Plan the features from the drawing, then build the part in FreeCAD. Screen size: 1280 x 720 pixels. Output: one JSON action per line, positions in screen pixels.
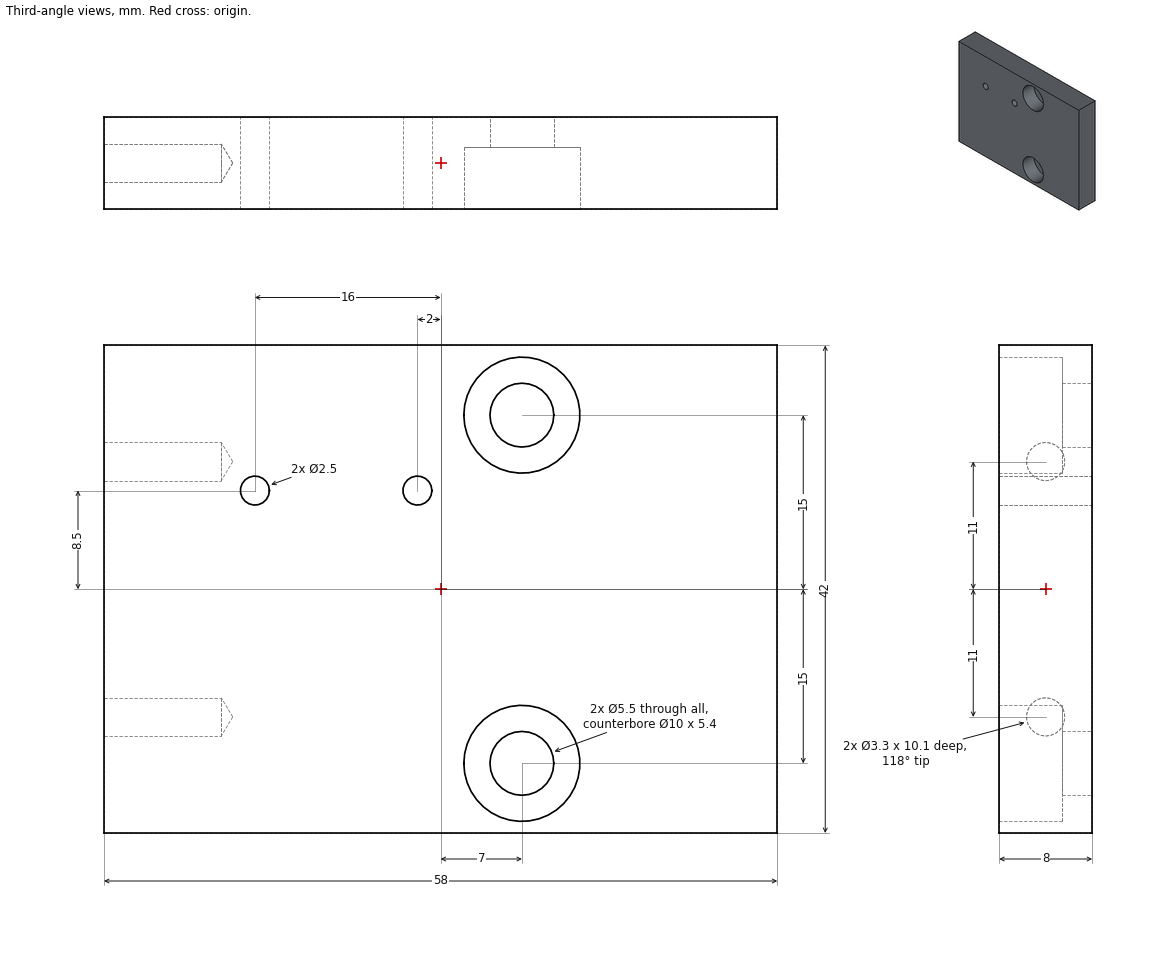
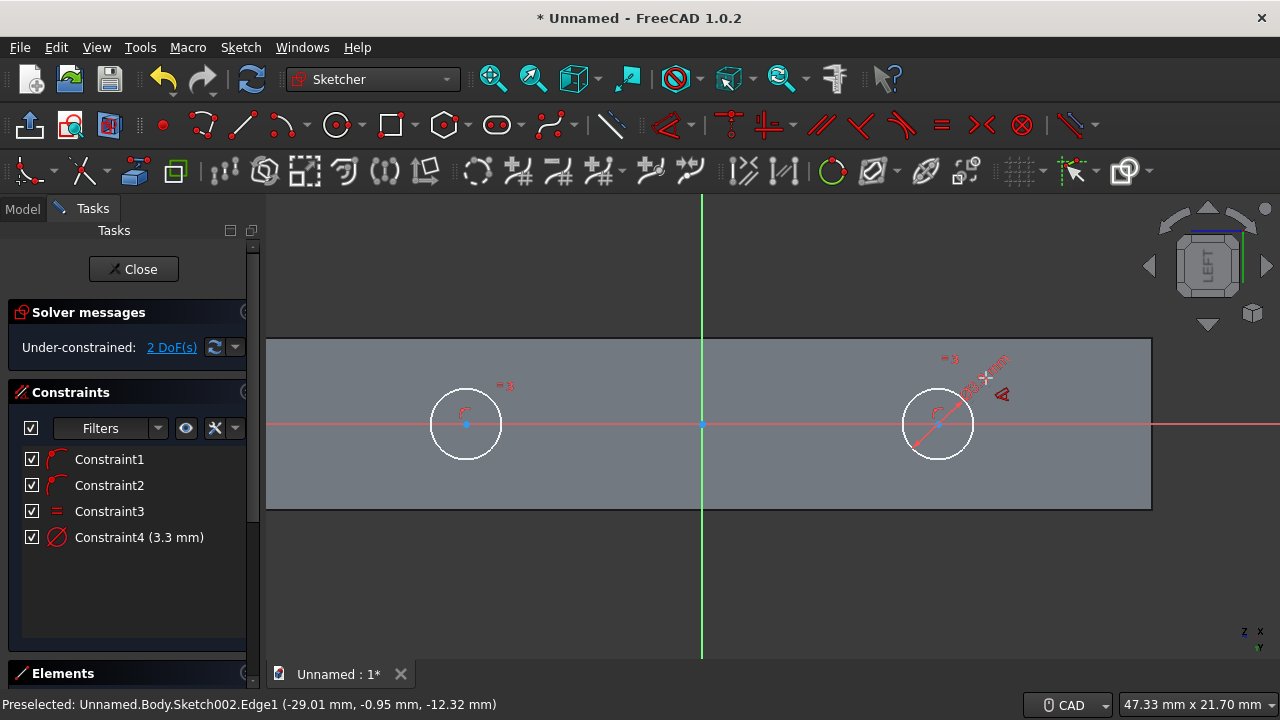
{"action": "left_click", "coordinate": [938, 424]}
{"action": "left_click", "coordinate": [820, 458]}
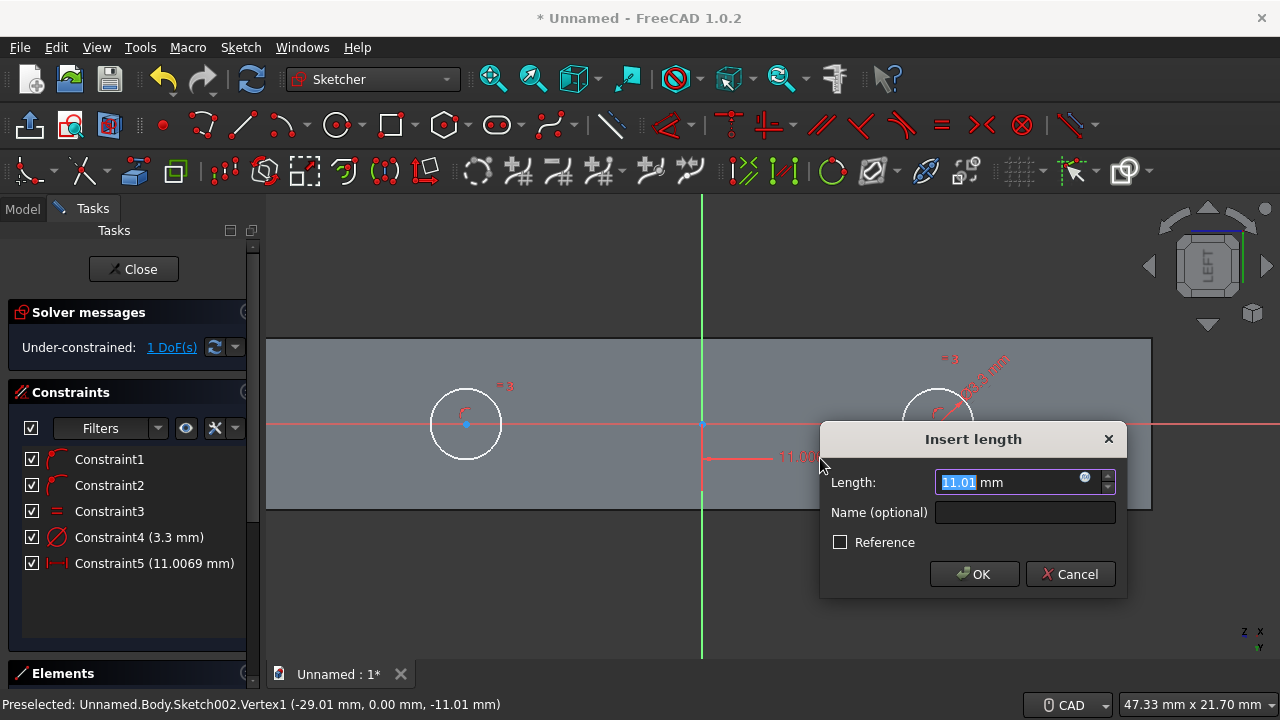
{"action": "type", "text": "11"}
{"action": "key", "text": "Return"}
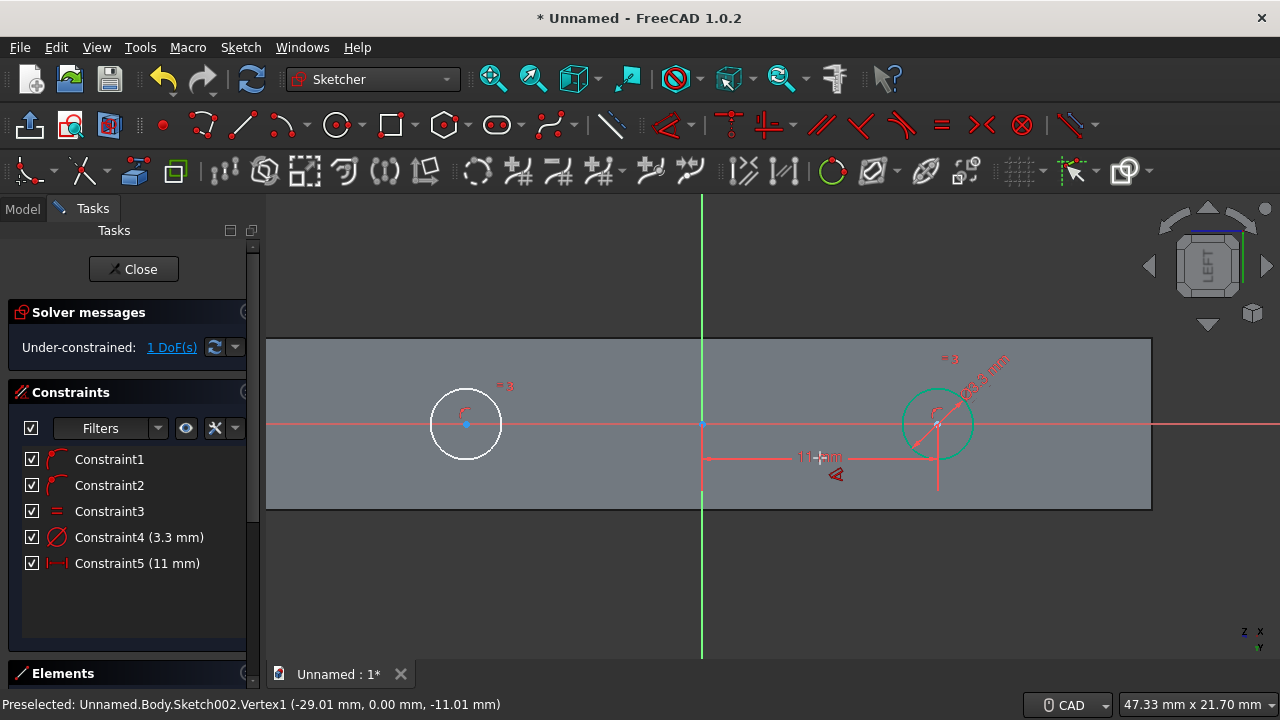
{"action": "left_click", "coordinate": [466, 424]}
{"action": "left_click", "coordinate": [584, 458]}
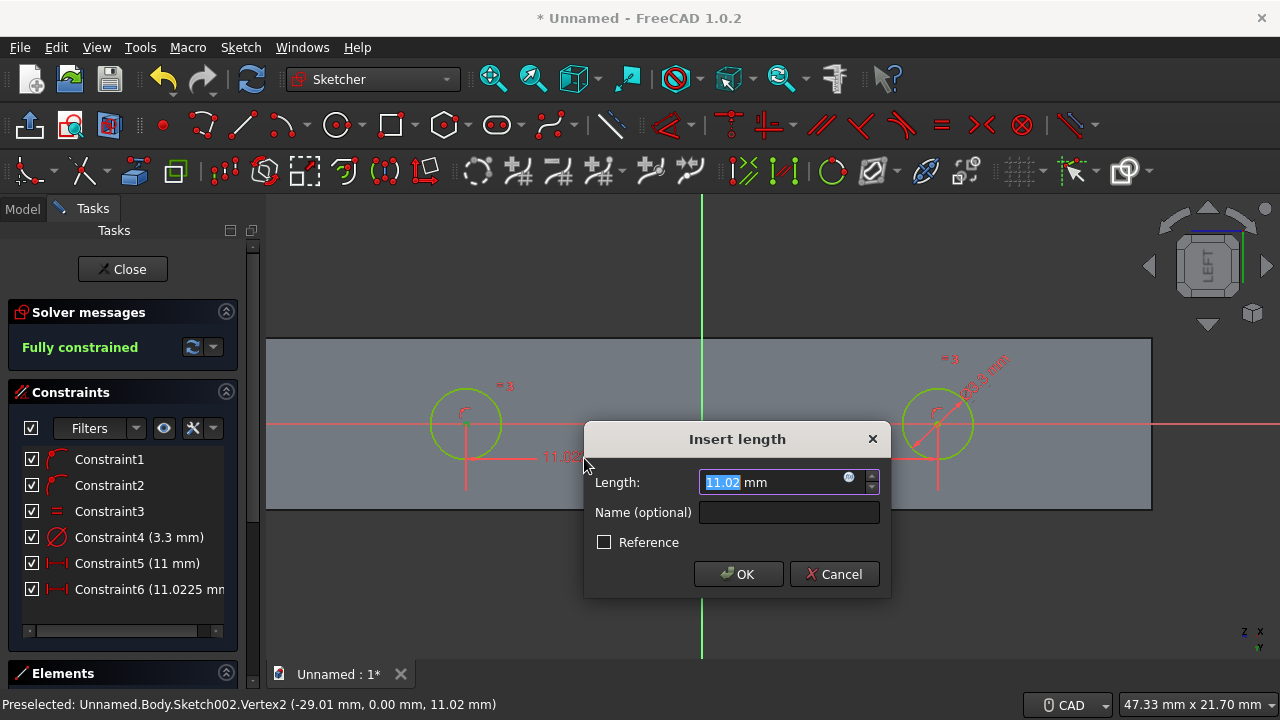
{"action": "type", "text": "11"}
{"action": "key", "text": "Return"}
{"action": "key", "text": "Escape"}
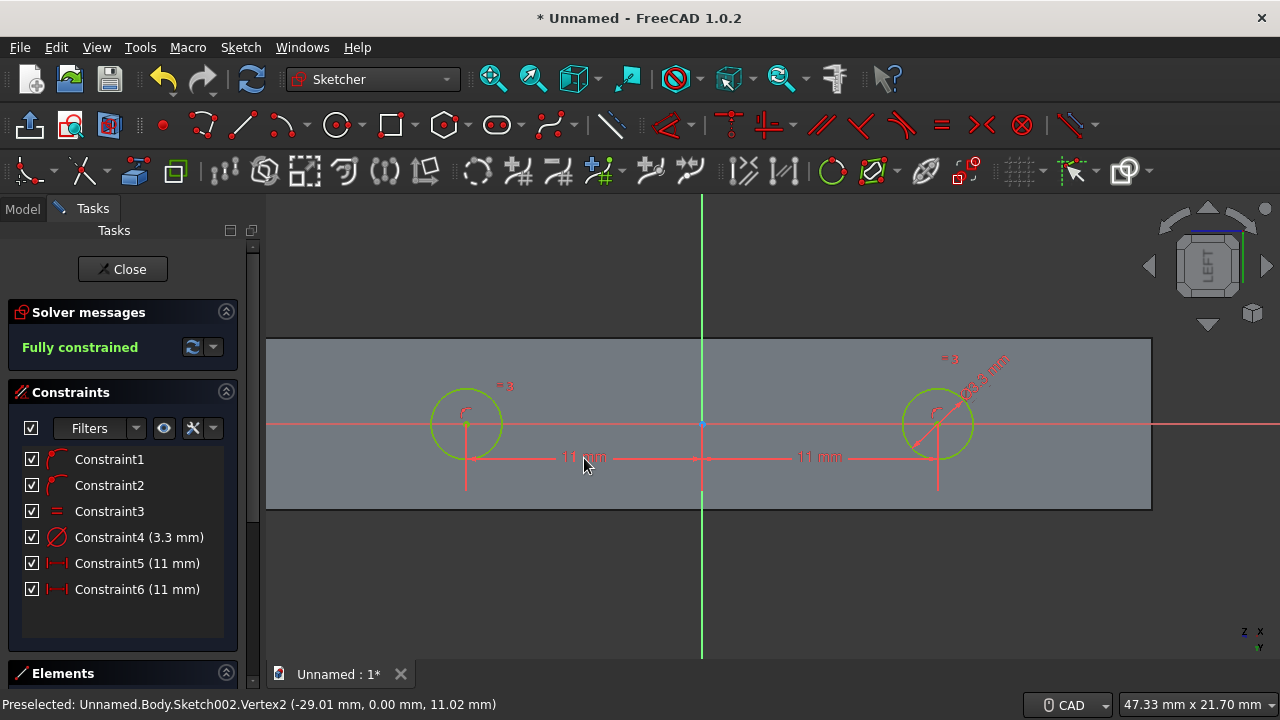
{"action": "left_click", "coordinate": [123, 269]}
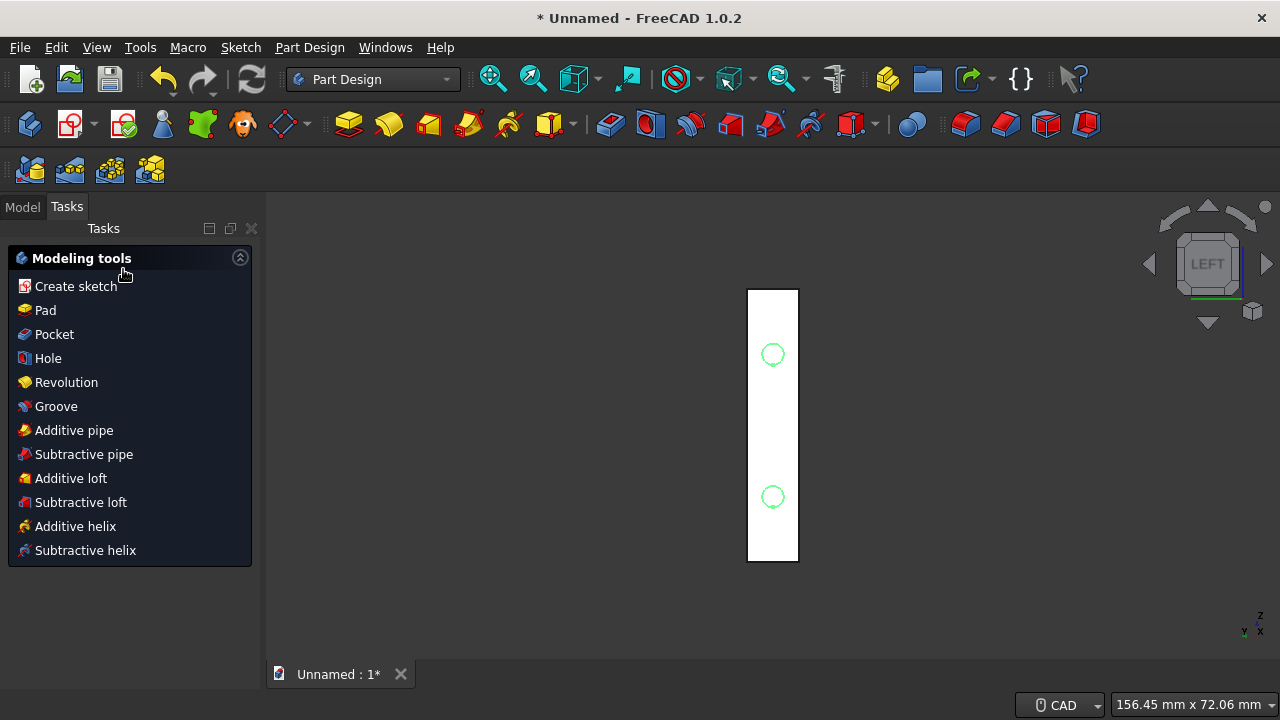
{"action": "left_click", "coordinate": [652, 124]}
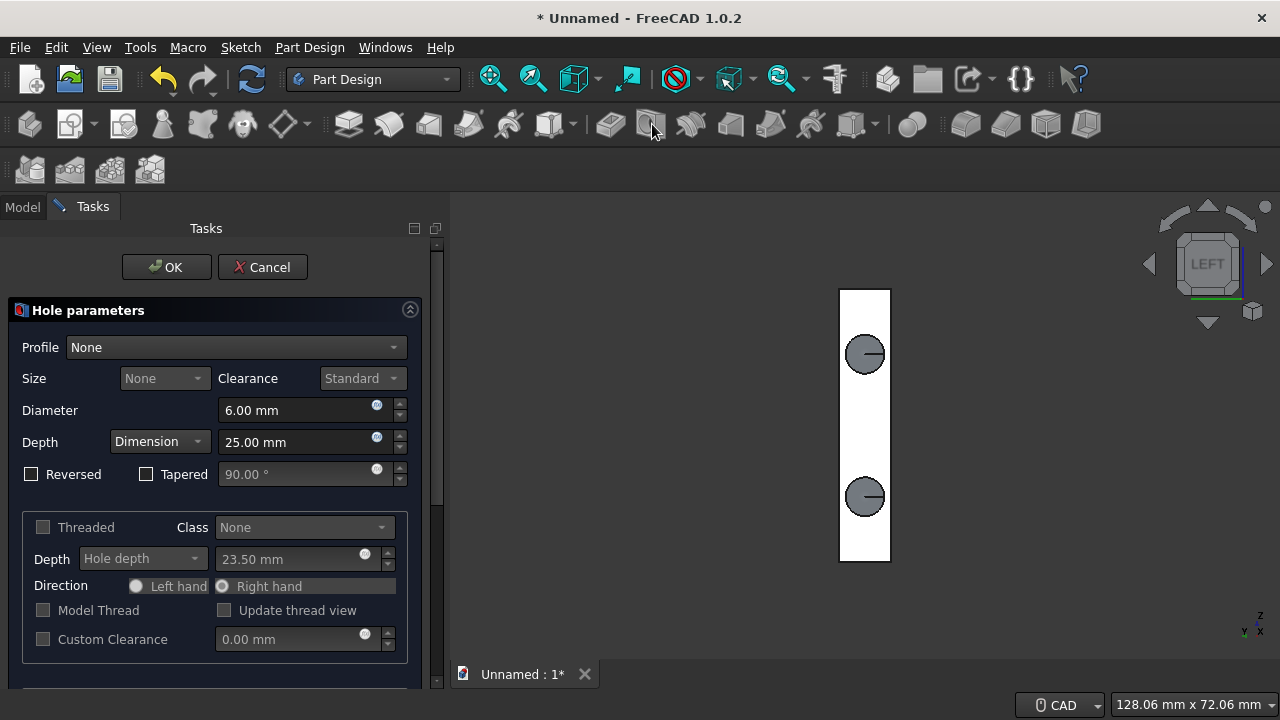
{"action": "triple_click", "coordinate": [305, 410]}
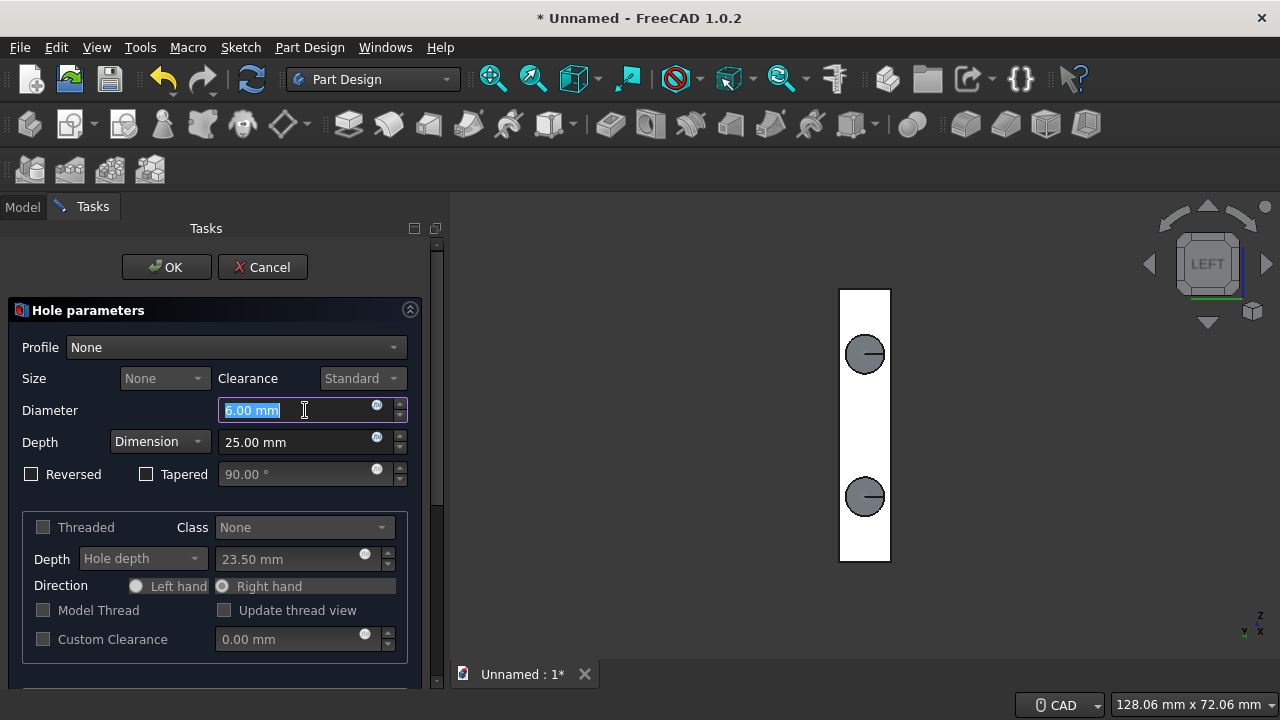
{"action": "type", "text": "3.3"}
{"action": "key", "text": "Tab"}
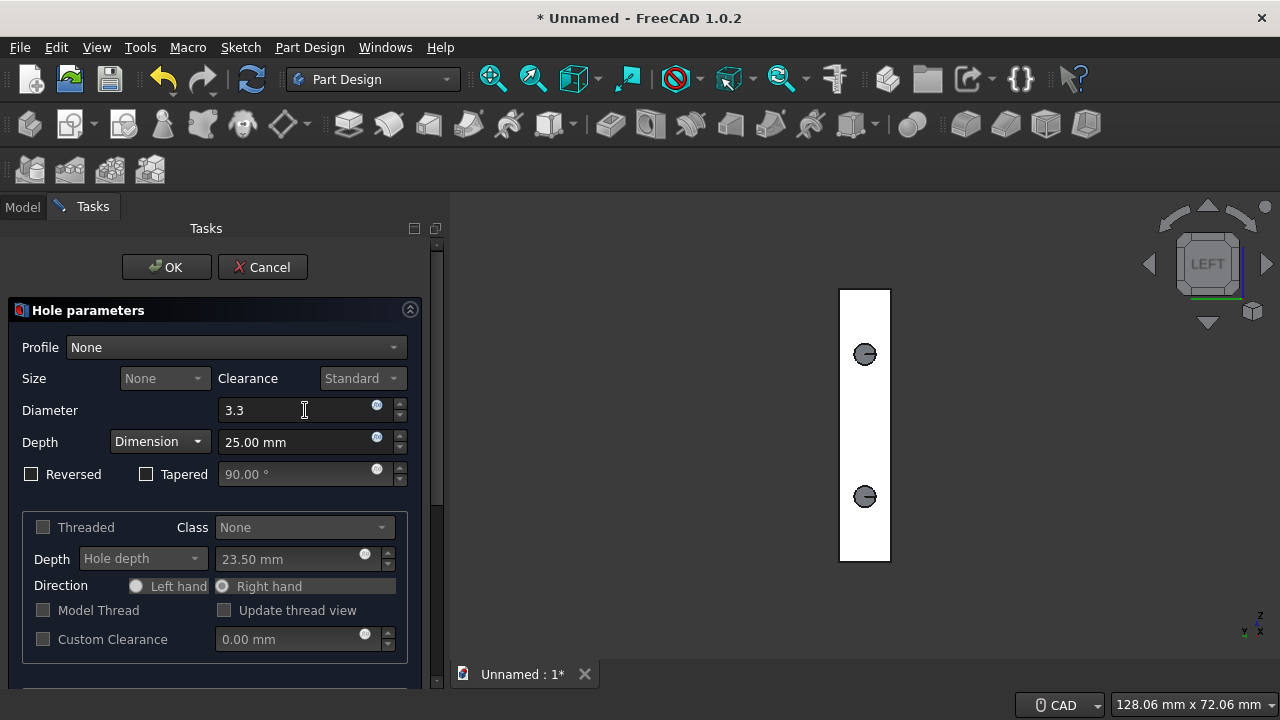
{"action": "triple_click", "coordinate": [305, 442]}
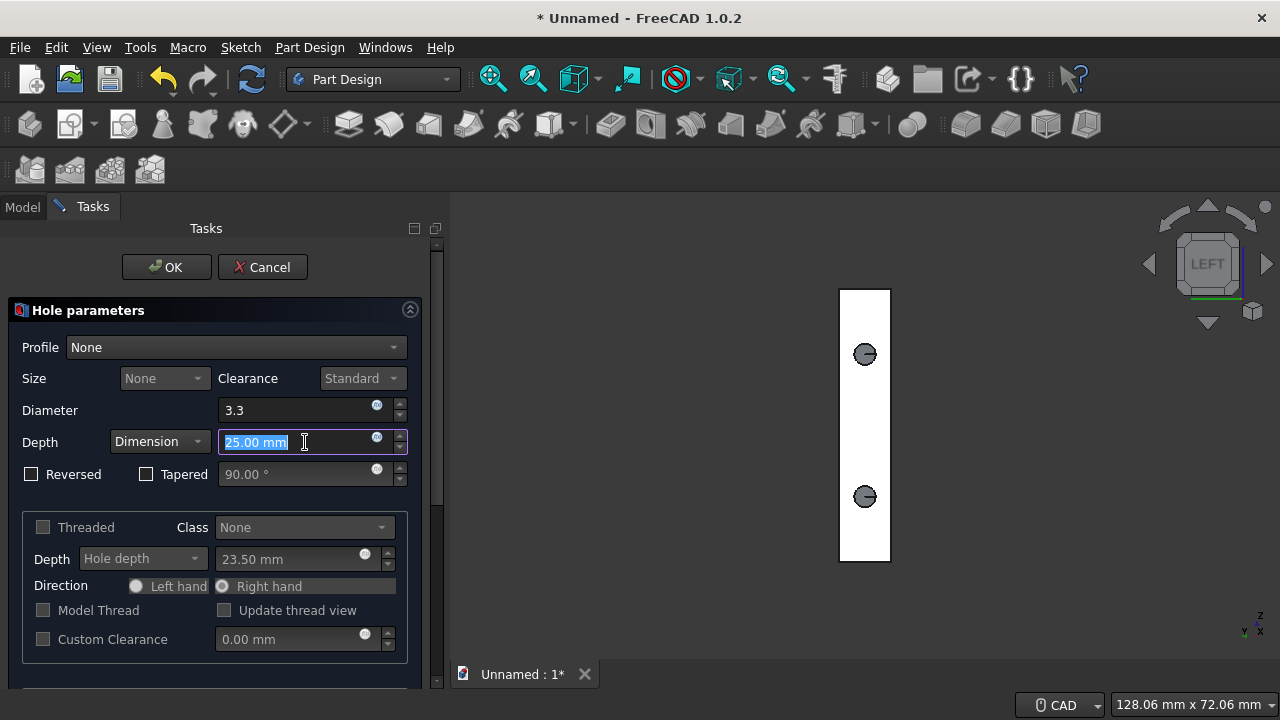
{"action": "type", "text": "10.1"}
{"action": "key", "text": "Tab"}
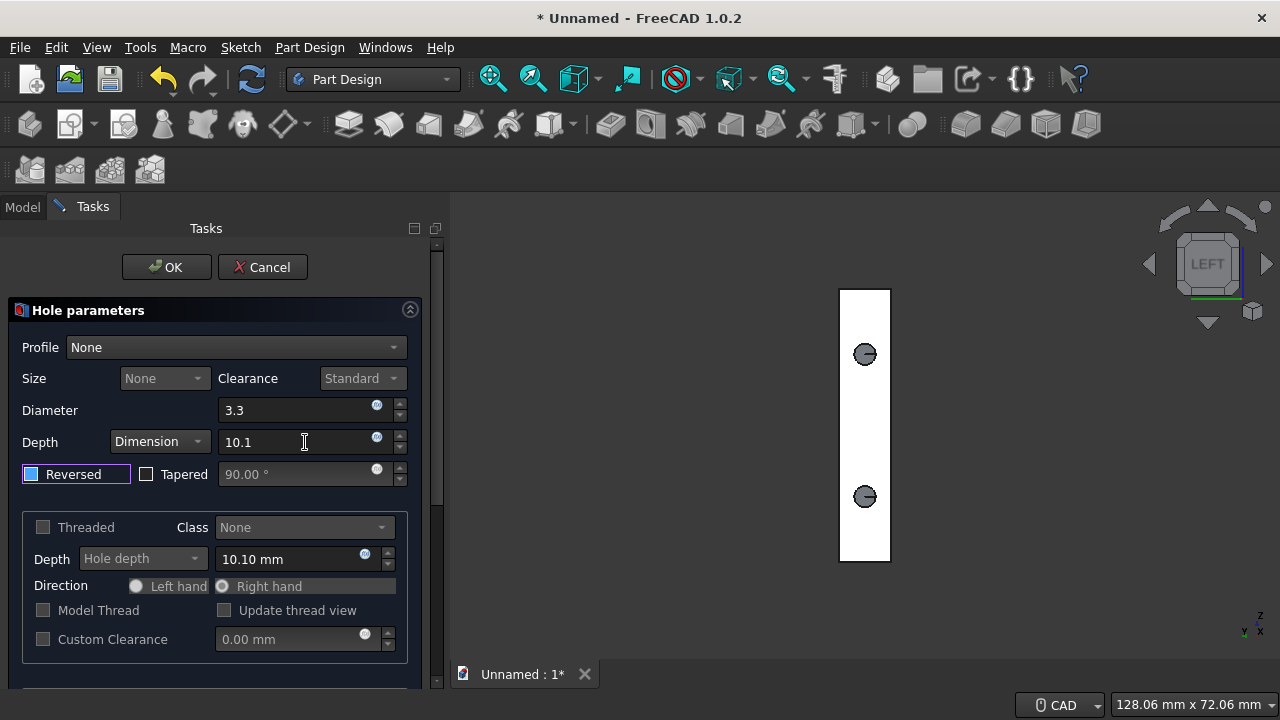
{"action": "left_click", "coordinate": [167, 267]}